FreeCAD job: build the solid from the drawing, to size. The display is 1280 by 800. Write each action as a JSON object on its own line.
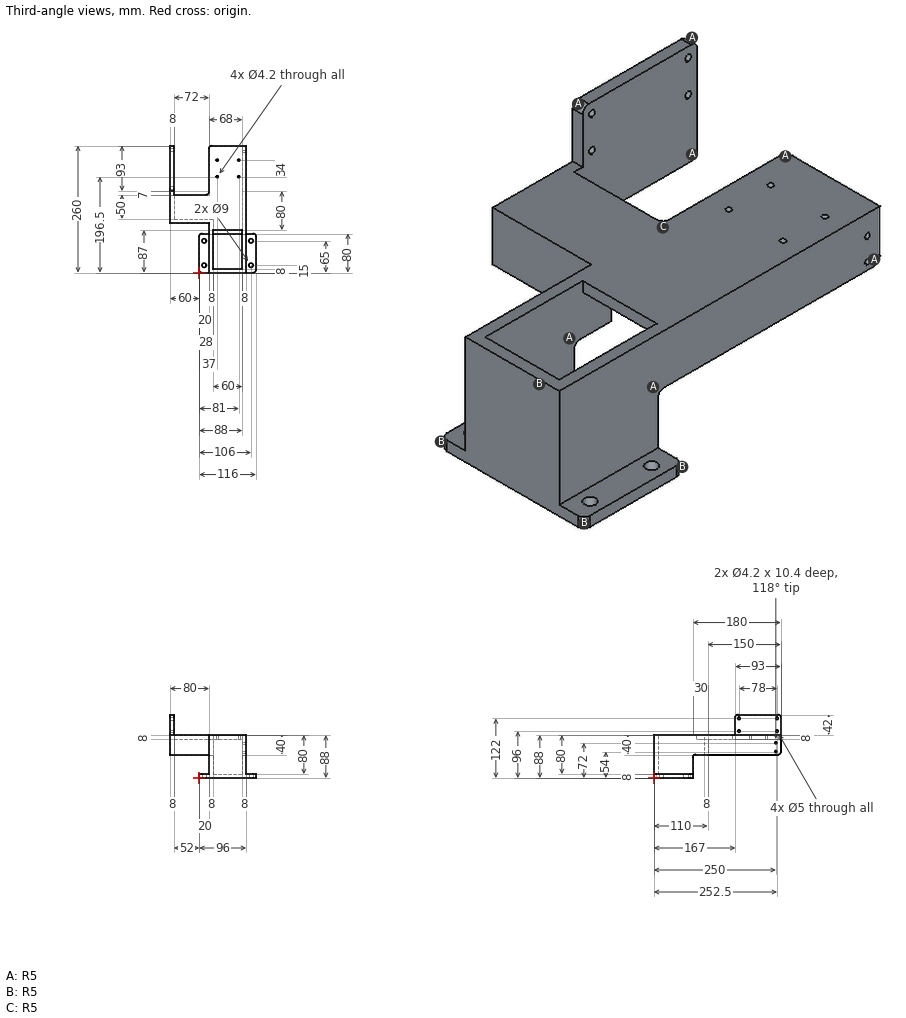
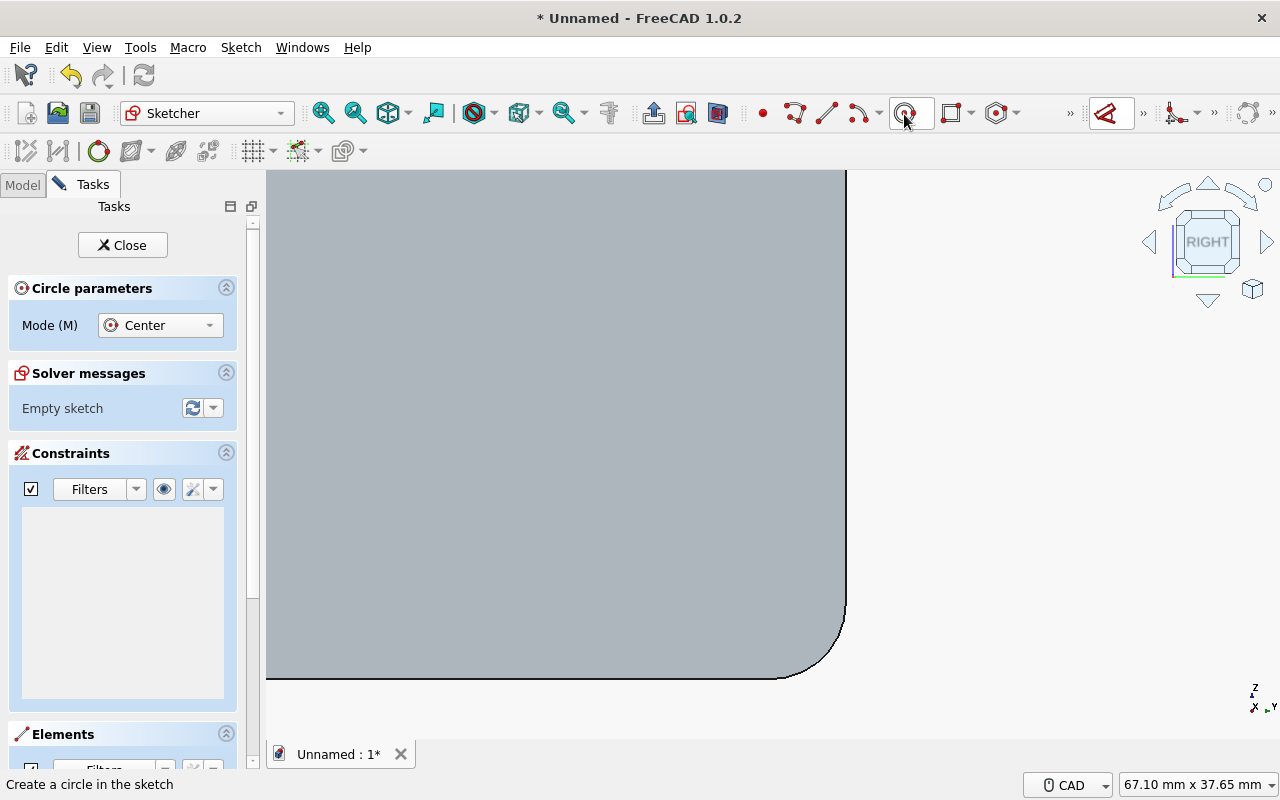
{"action": "left_click", "coordinate": [695, 317]}
{"action": "left_click", "coordinate": [717, 294]}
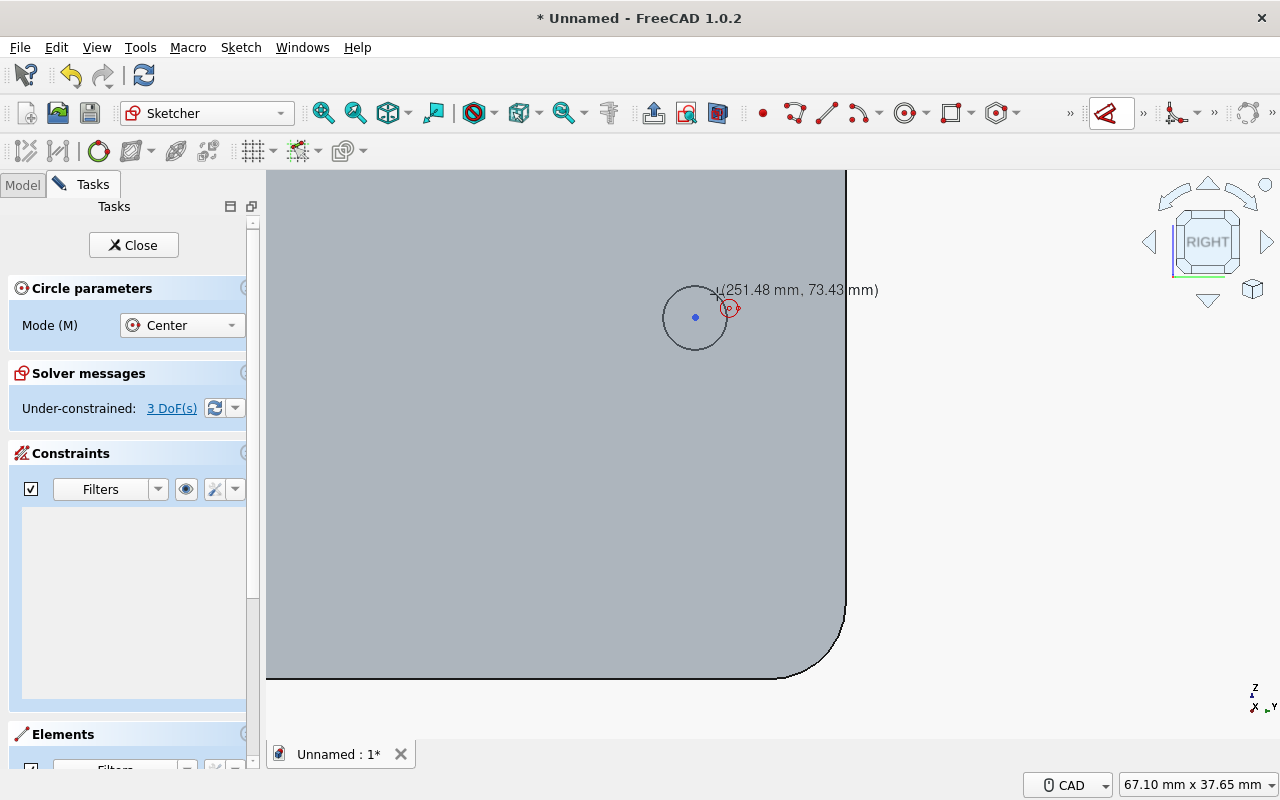
{"action": "left_click", "coordinate": [695, 589]}
{"action": "left_click", "coordinate": [717, 566]}
{"action": "key", "text": "Escape"}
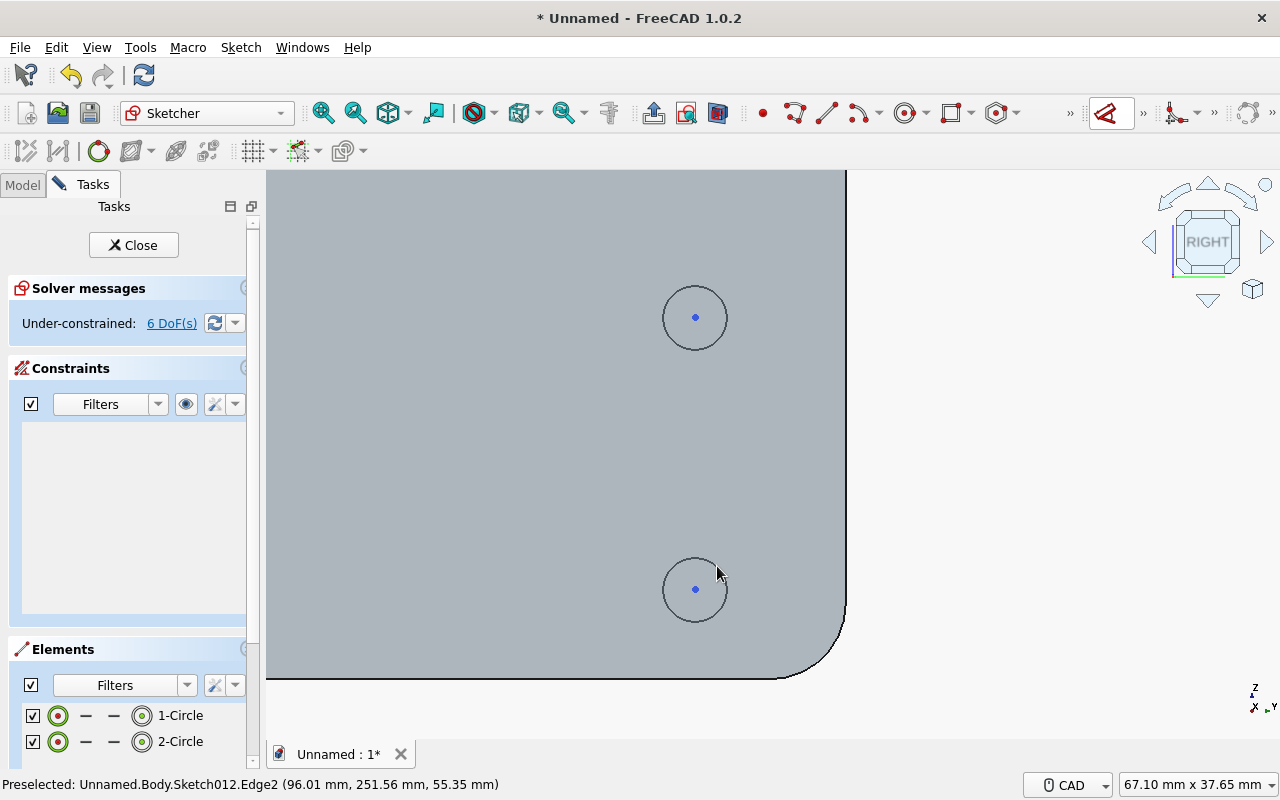
{"action": "left_click", "coordinate": [717, 295]}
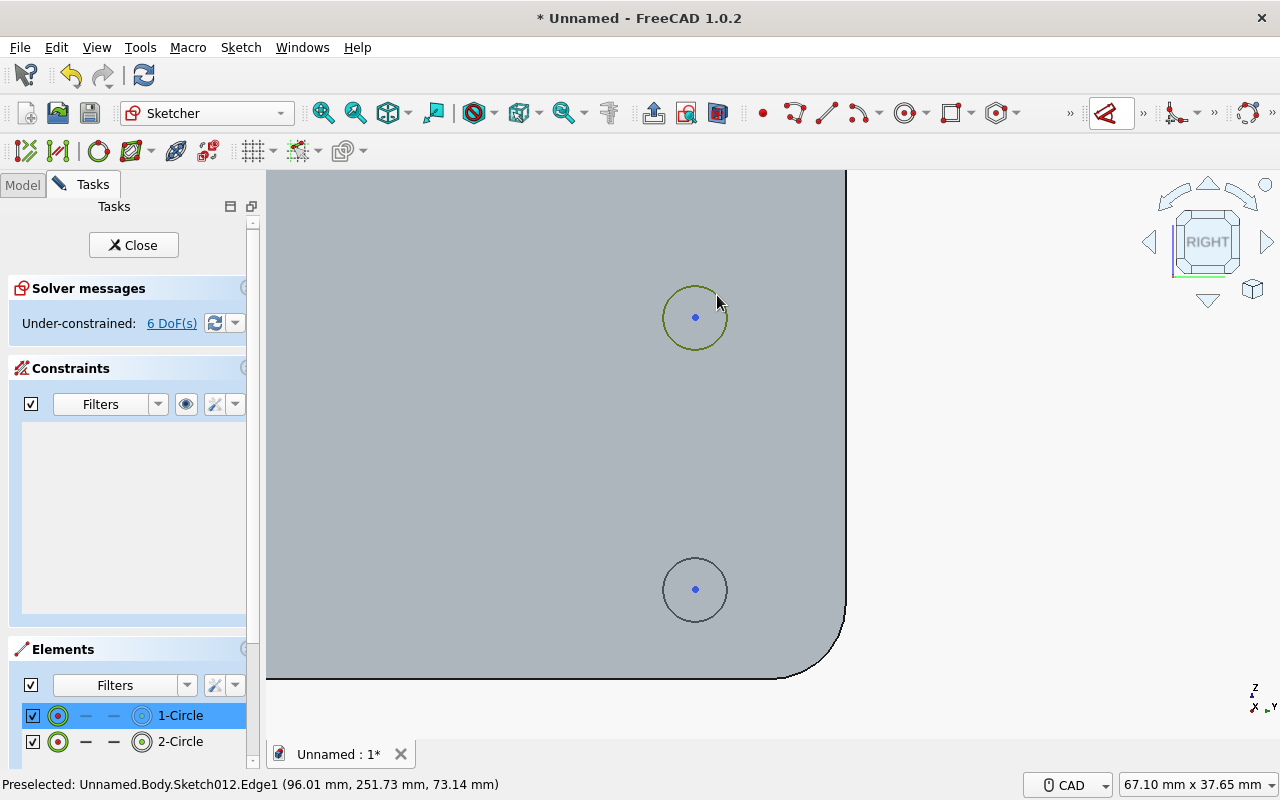
{"action": "left_click", "coordinate": [717, 567]}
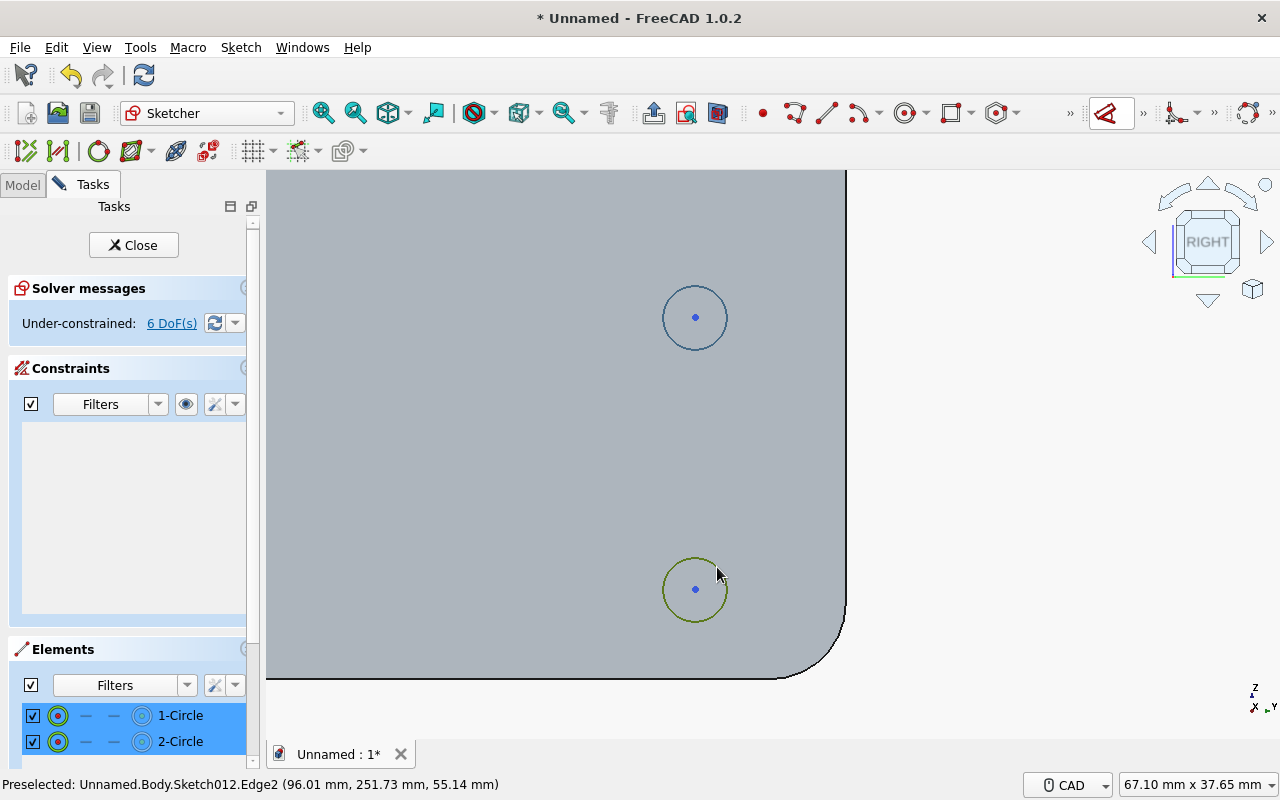
{"action": "key", "text": "e"}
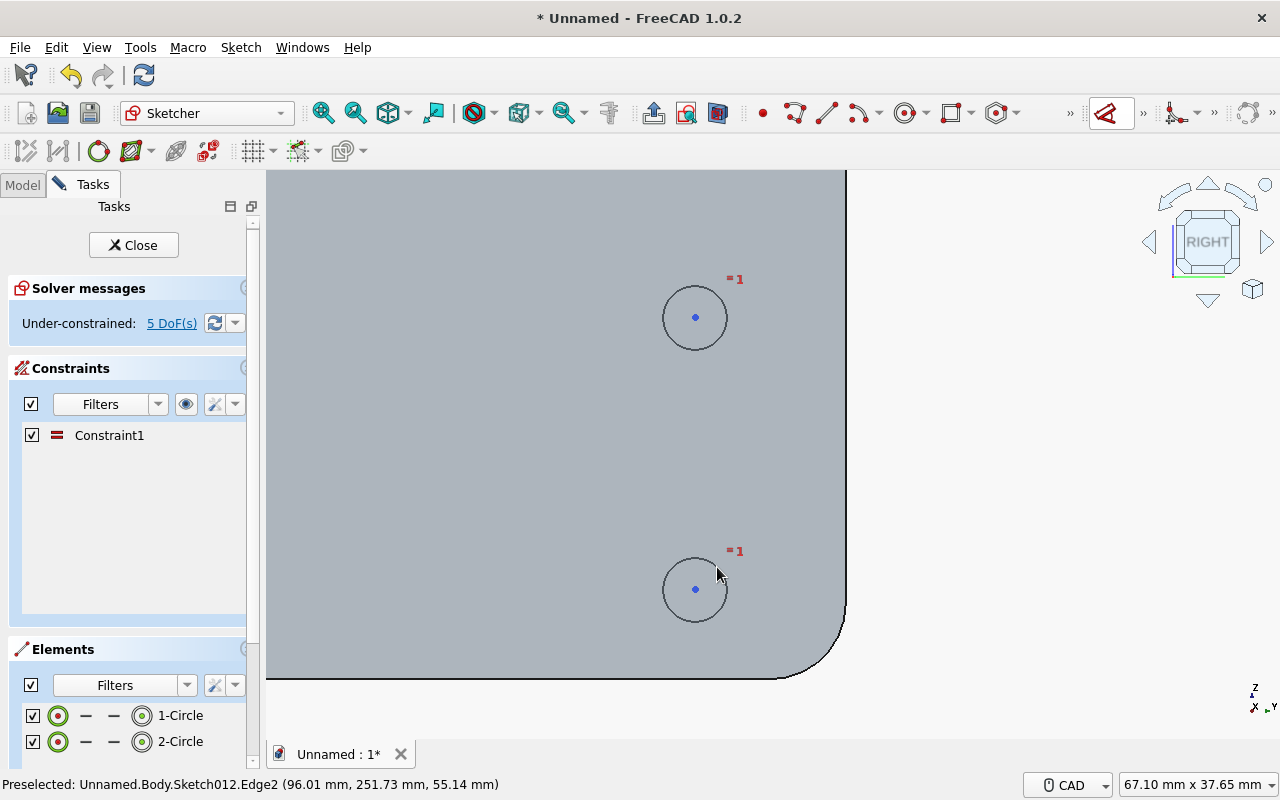
{"action": "left_click", "coordinate": [695, 318]}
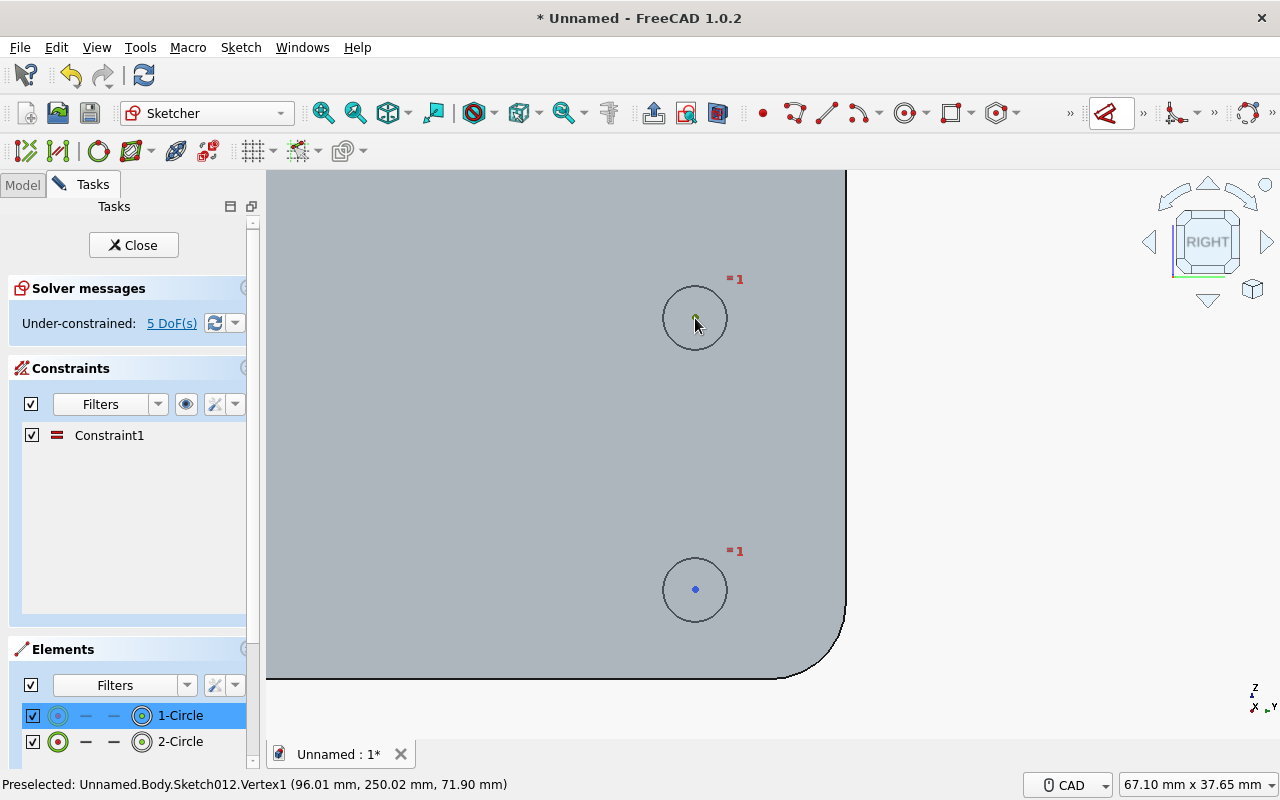
{"action": "left_click", "coordinate": [695, 590]}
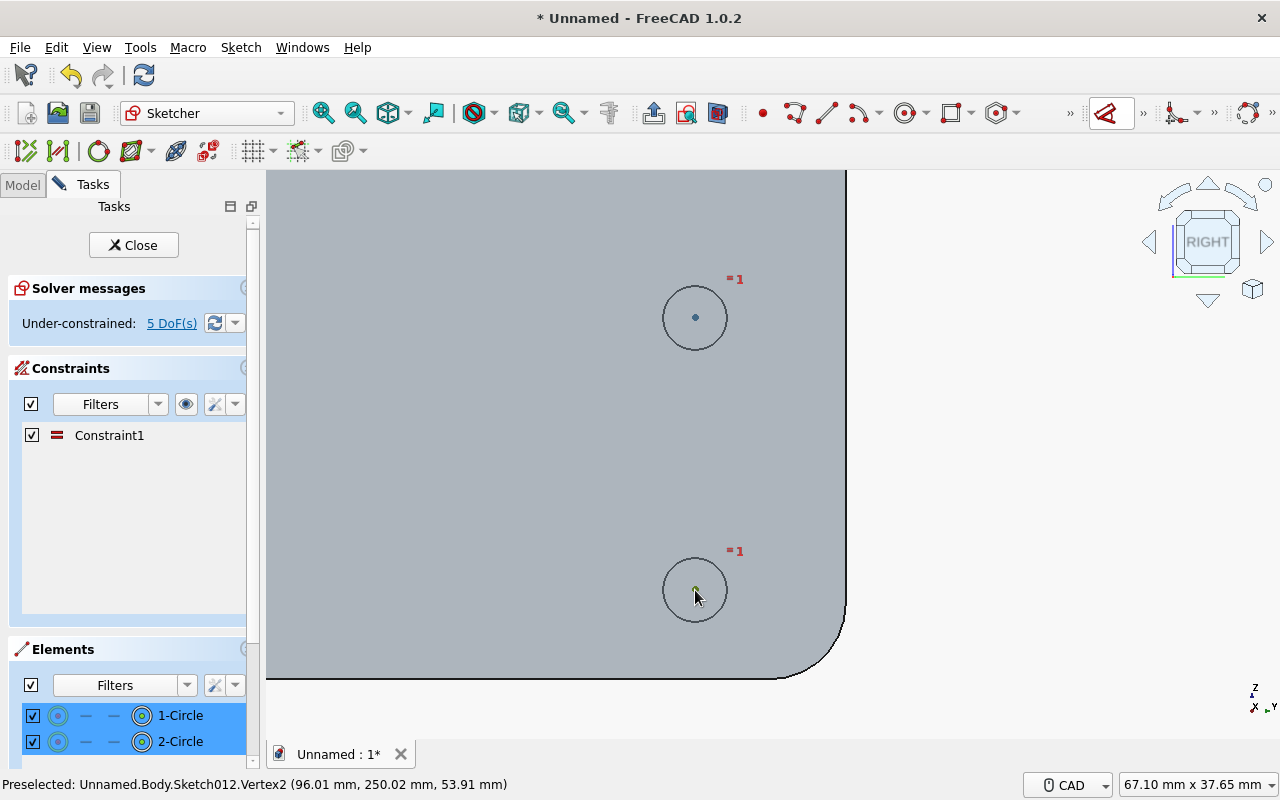
{"action": "key", "text": "v"}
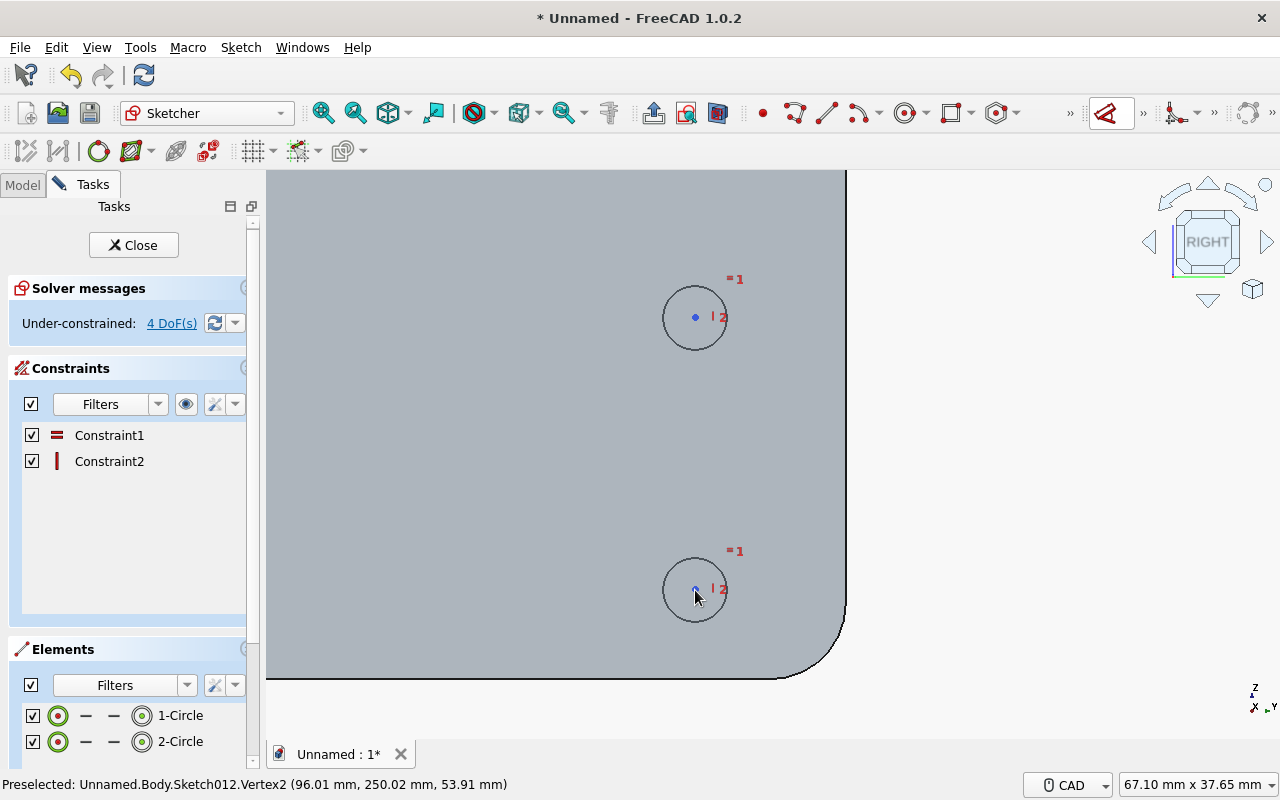
{"action": "left_click", "coordinate": [717, 295]}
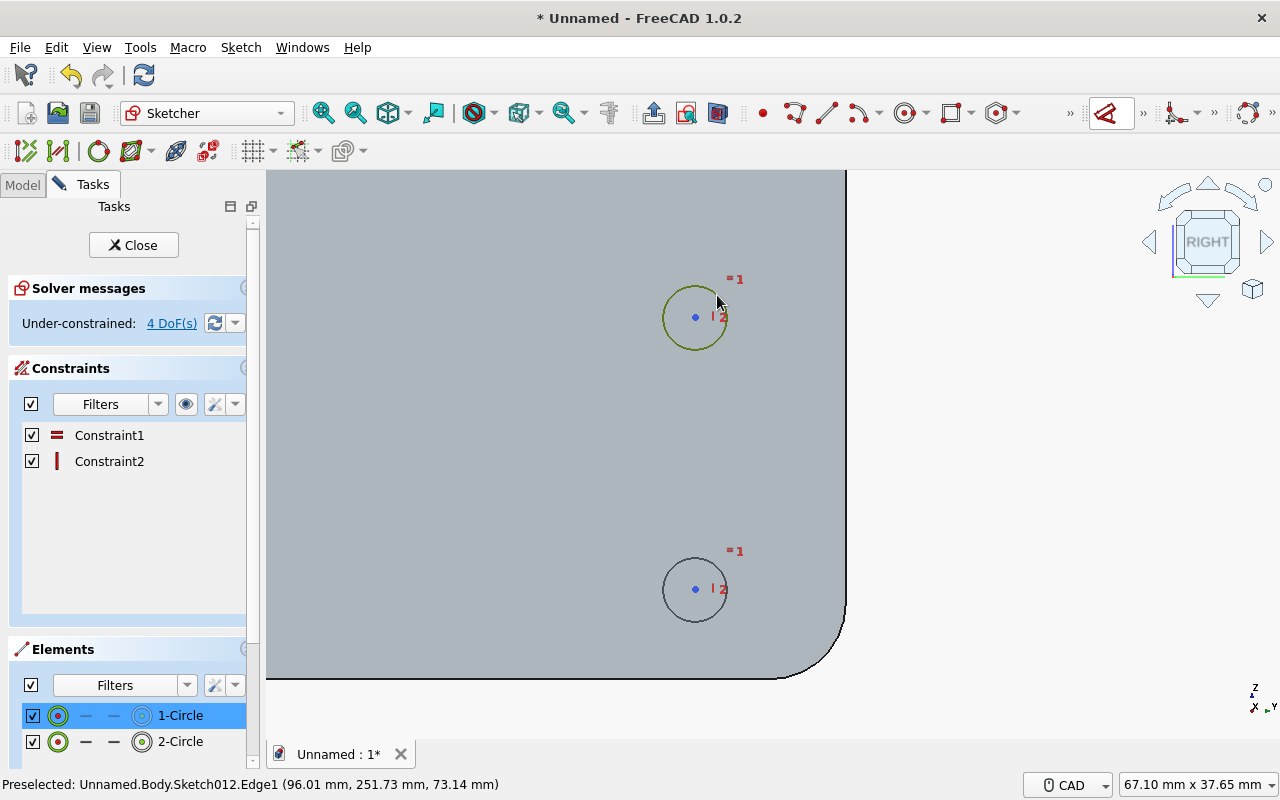
{"action": "left_click", "coordinate": [1128, 114]}